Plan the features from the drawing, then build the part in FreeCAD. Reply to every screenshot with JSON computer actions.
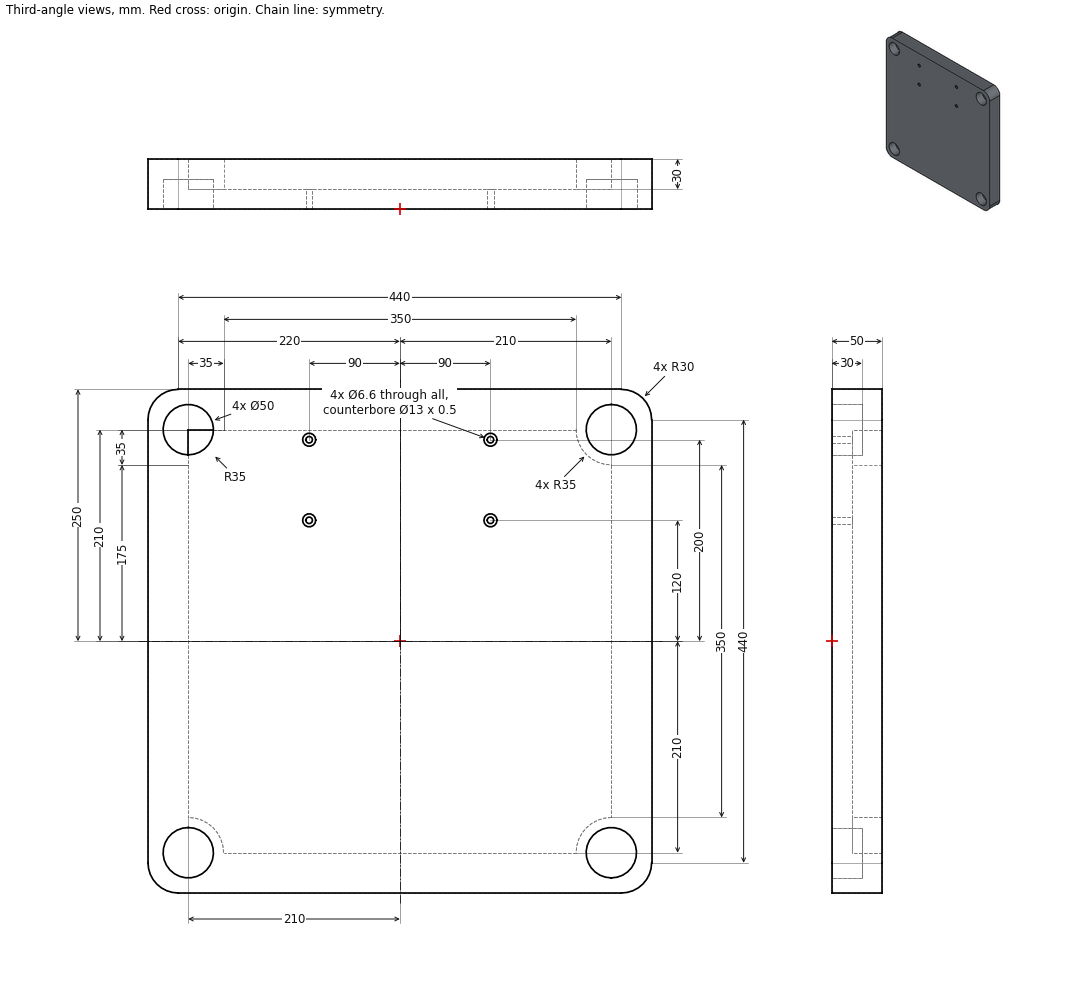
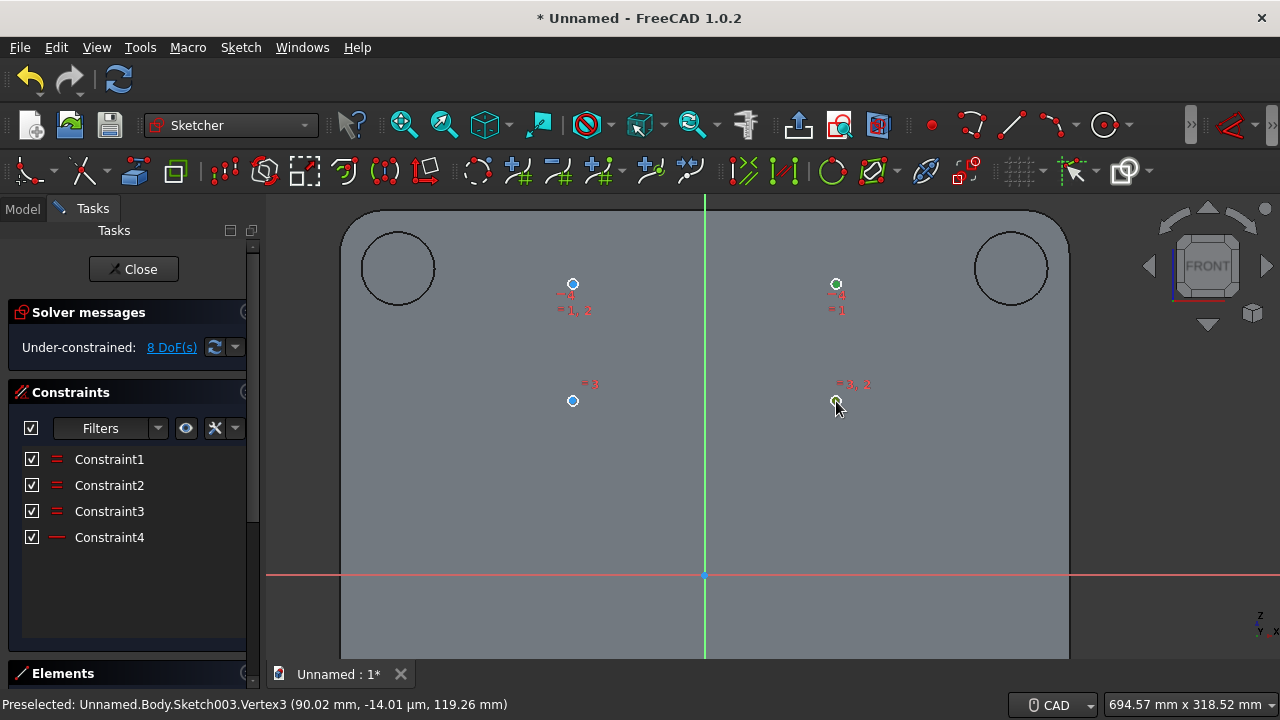
{"action": "key", "text": "v"}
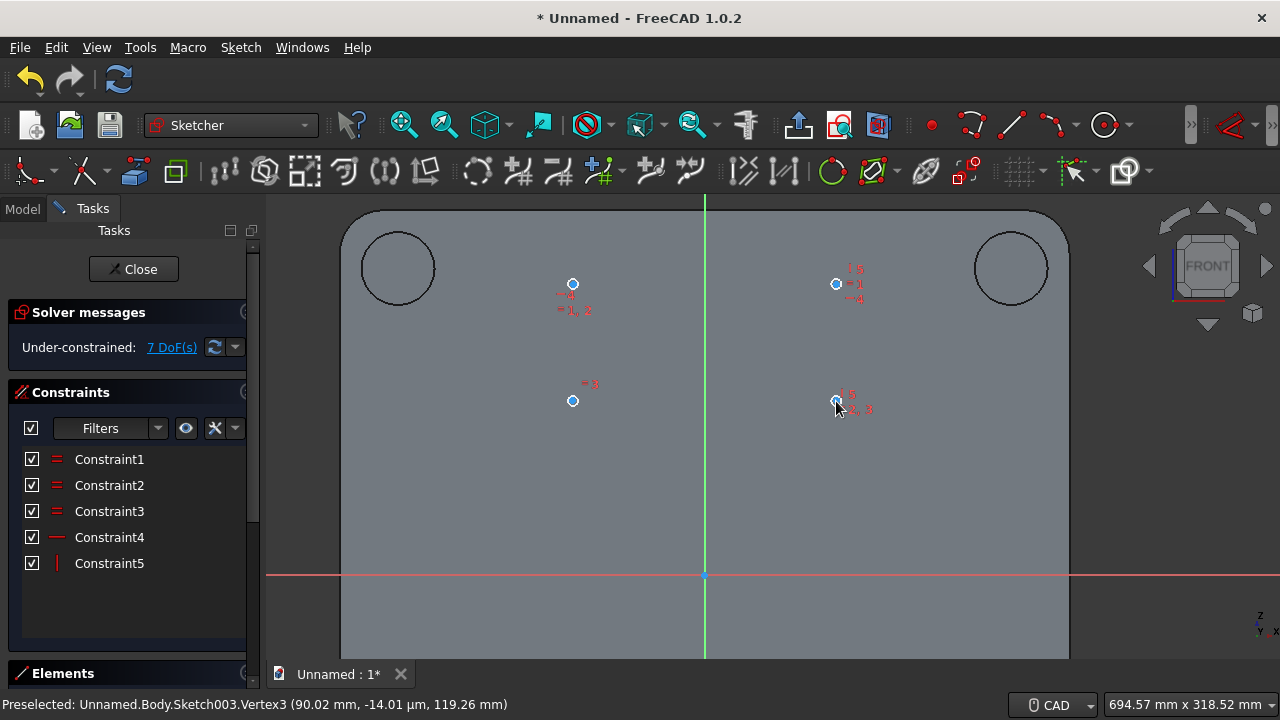
{"action": "left_click", "coordinate": [573, 284]}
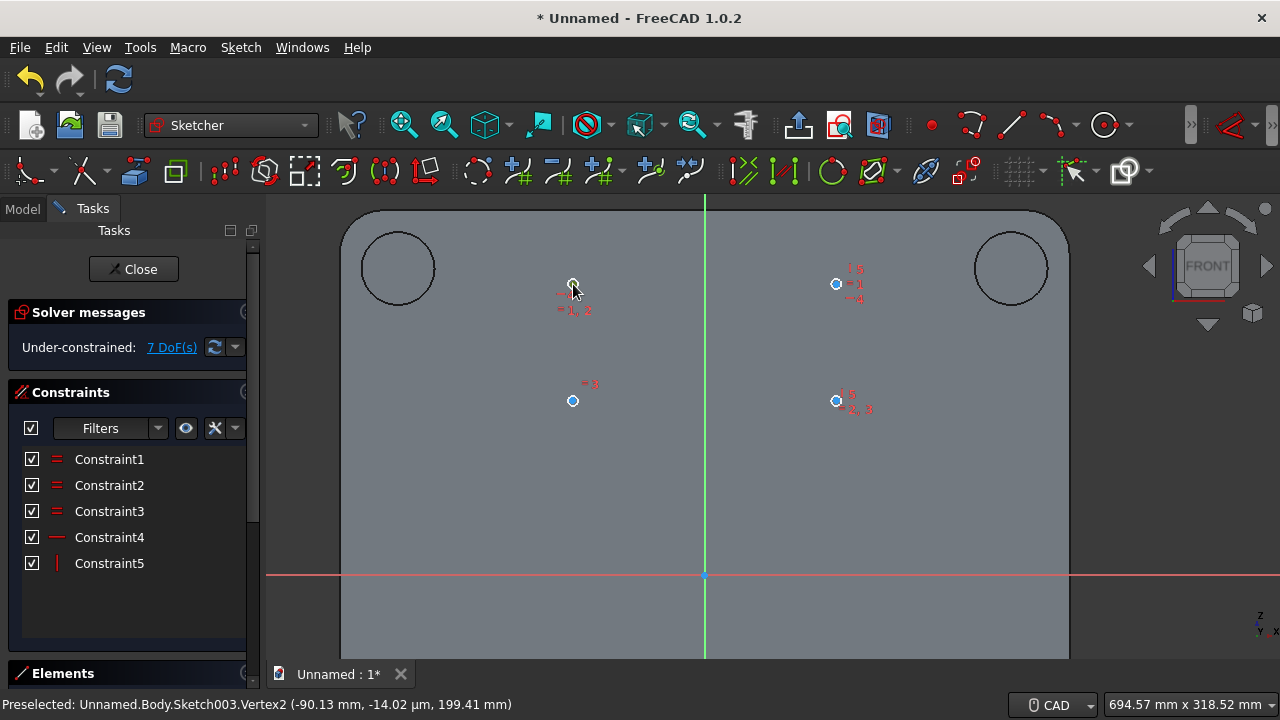
{"action": "left_click", "coordinate": [573, 401]}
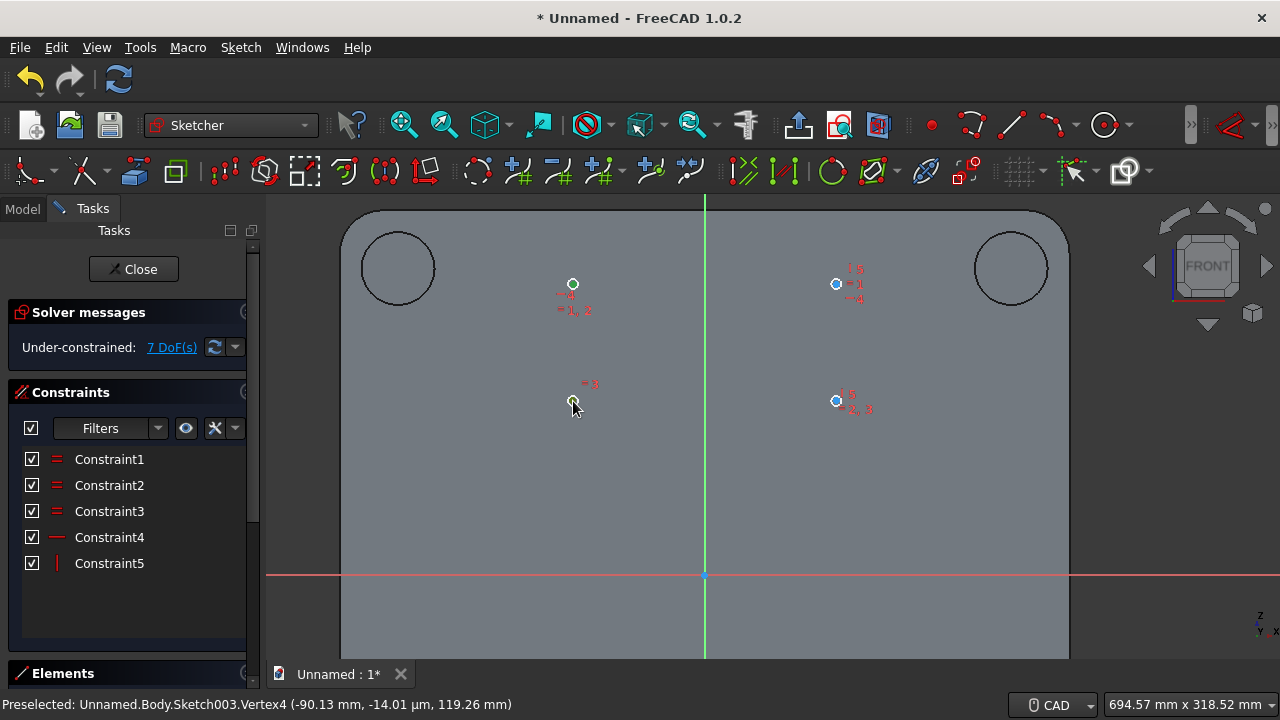
{"action": "key", "text": "v"}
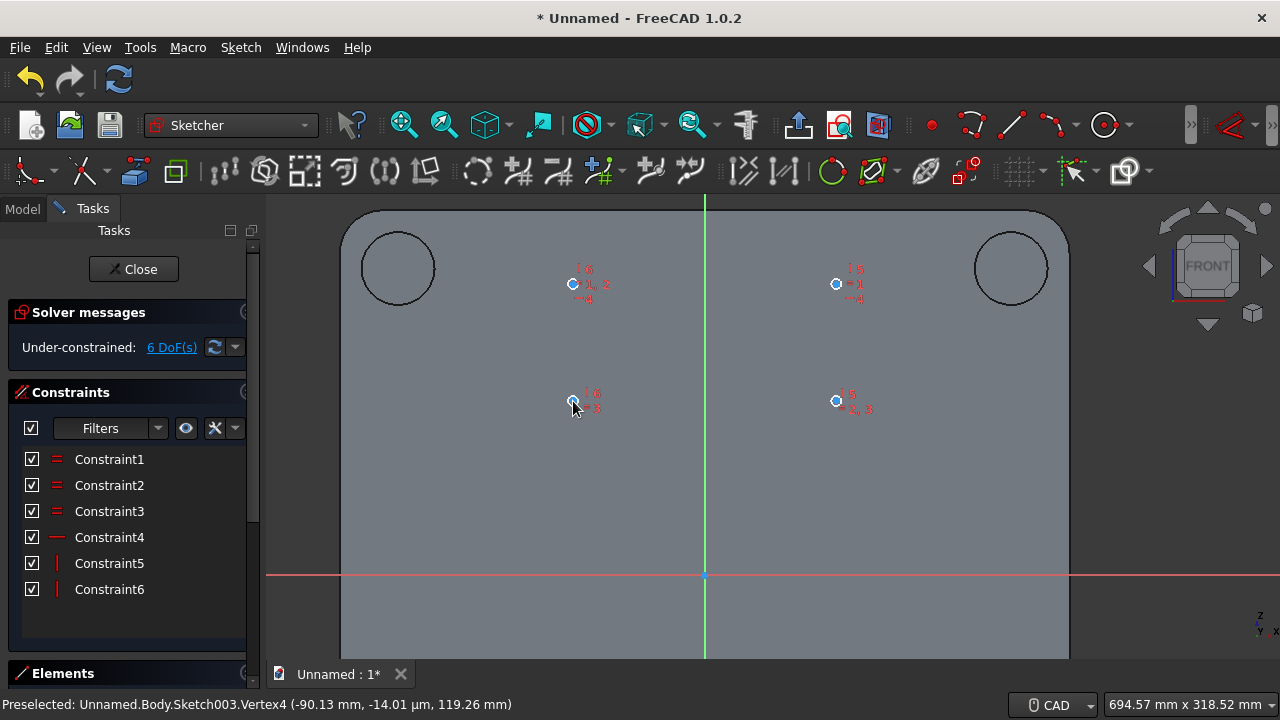
{"action": "left_click", "coordinate": [836, 401]}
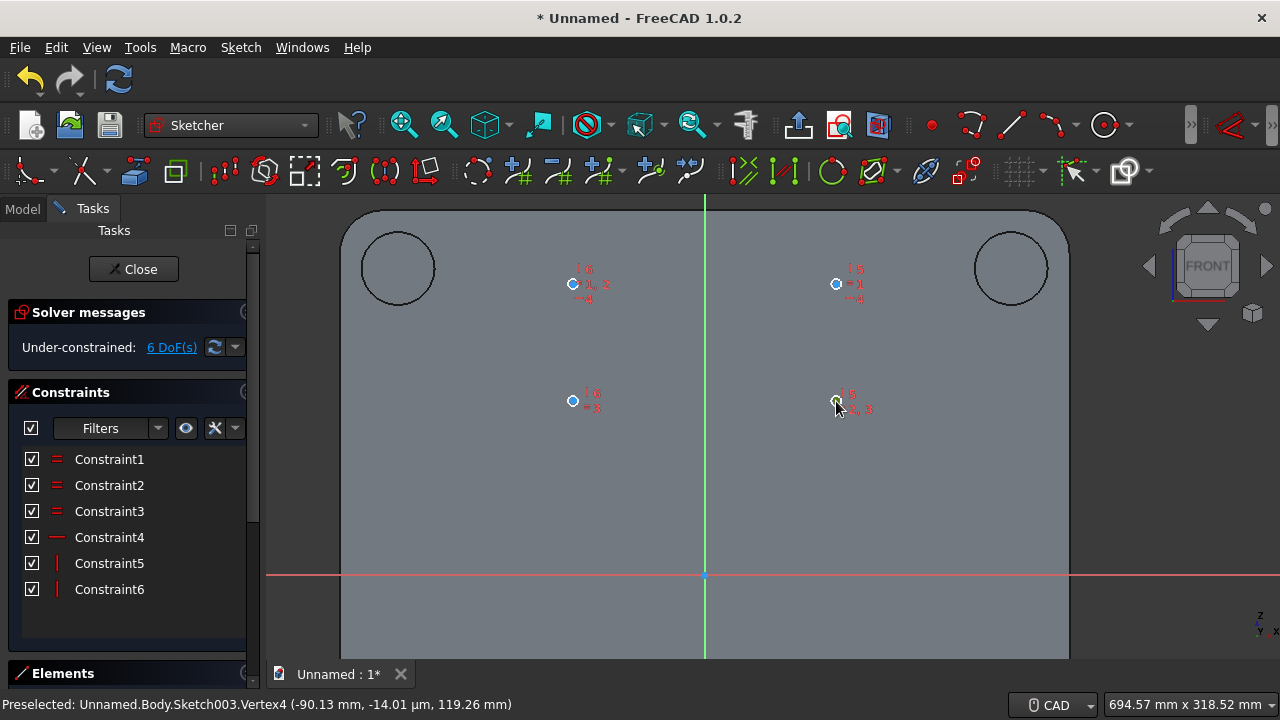
{"action": "left_click", "coordinate": [573, 401]}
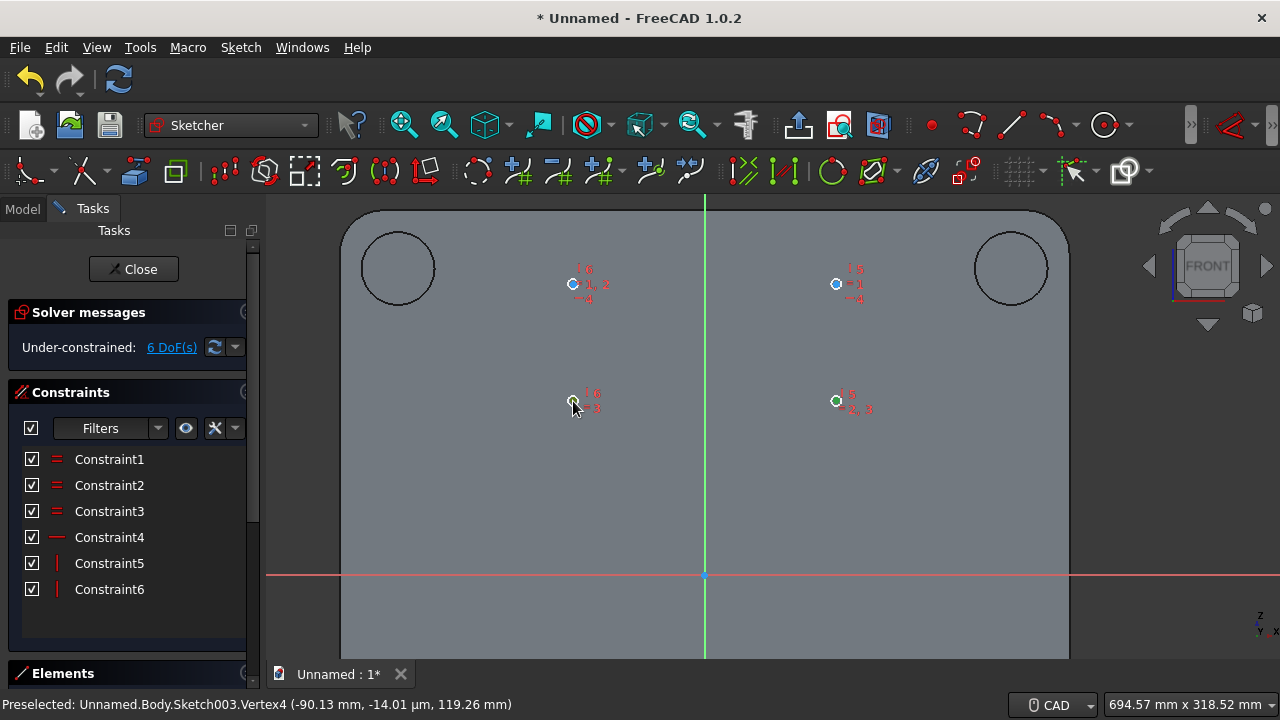
{"action": "key", "text": "h"}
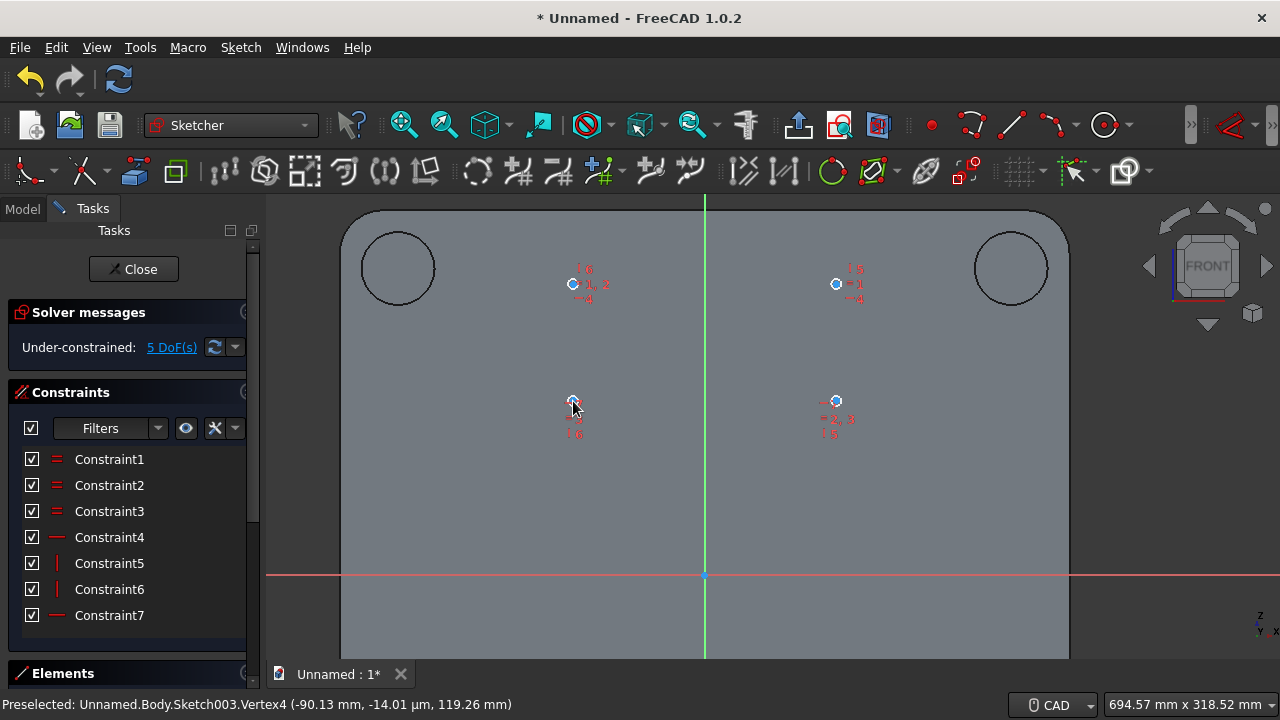
{"action": "key", "text": "d"}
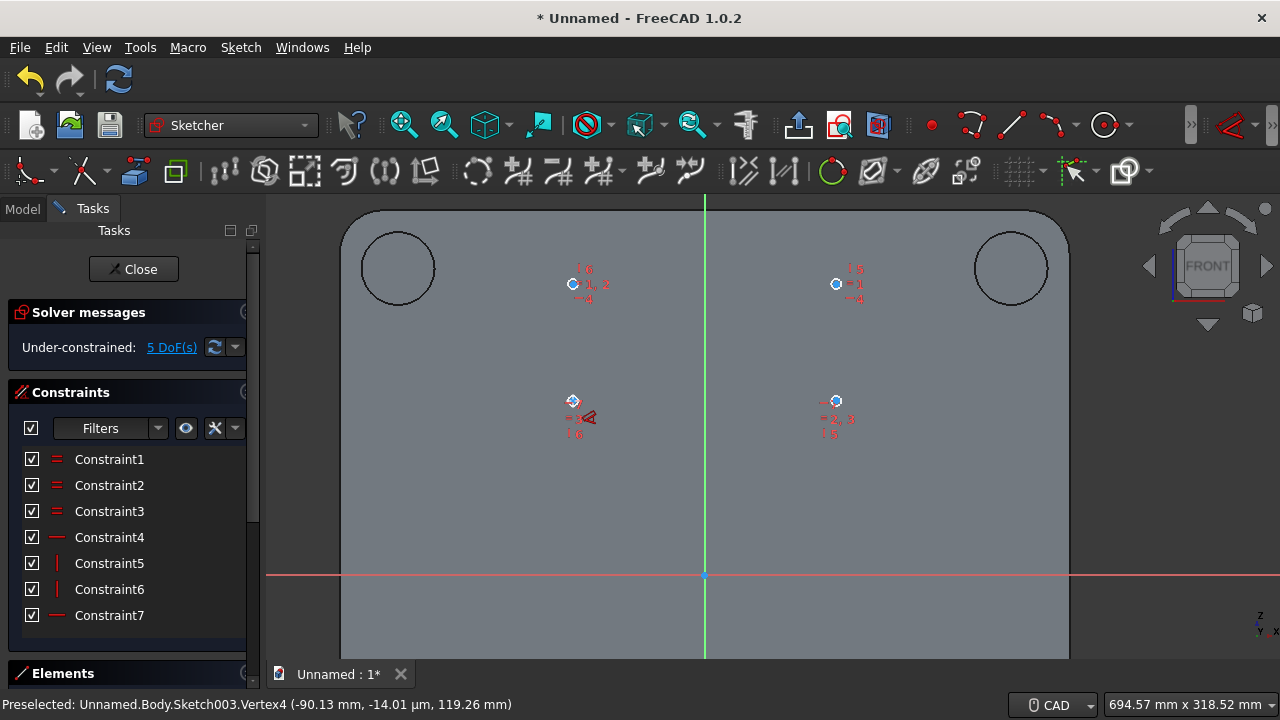
{"action": "scroll", "coordinate": [836, 279], "scroll_direction": "up", "scroll_amount": 8}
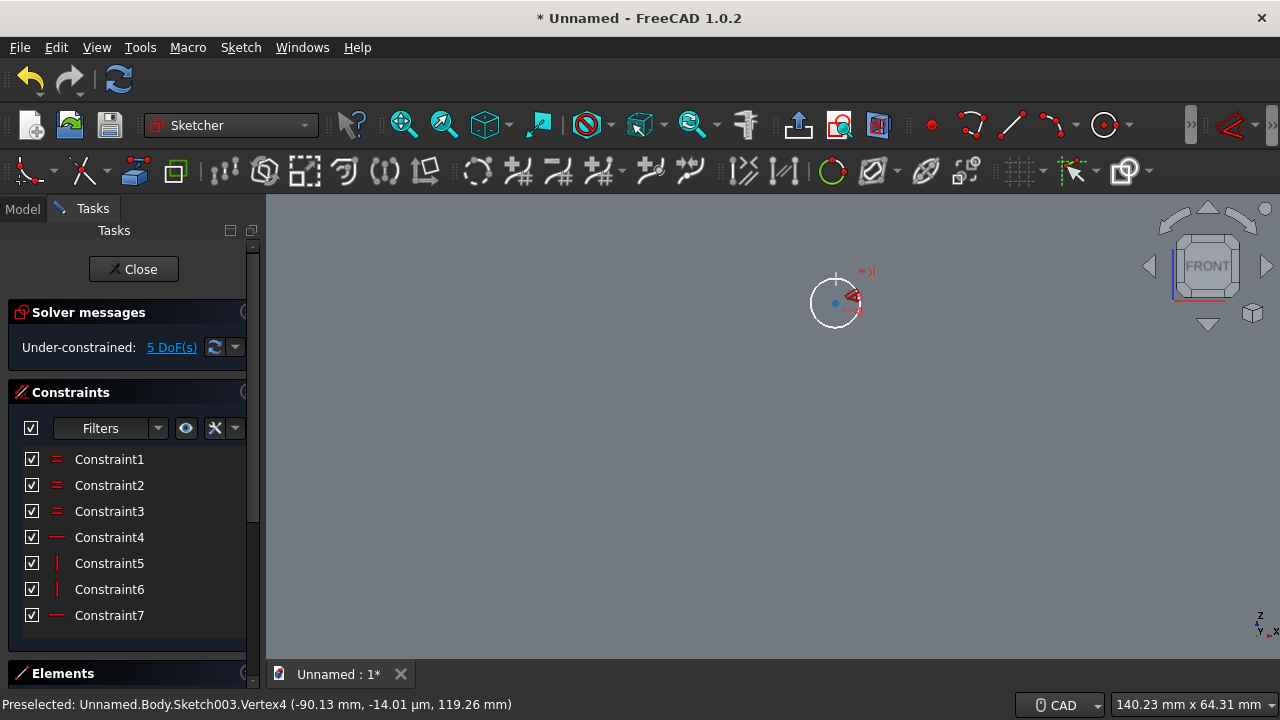
{"action": "left_click", "coordinate": [836, 279]}
{"action": "left_click", "coordinate": [837, 247]}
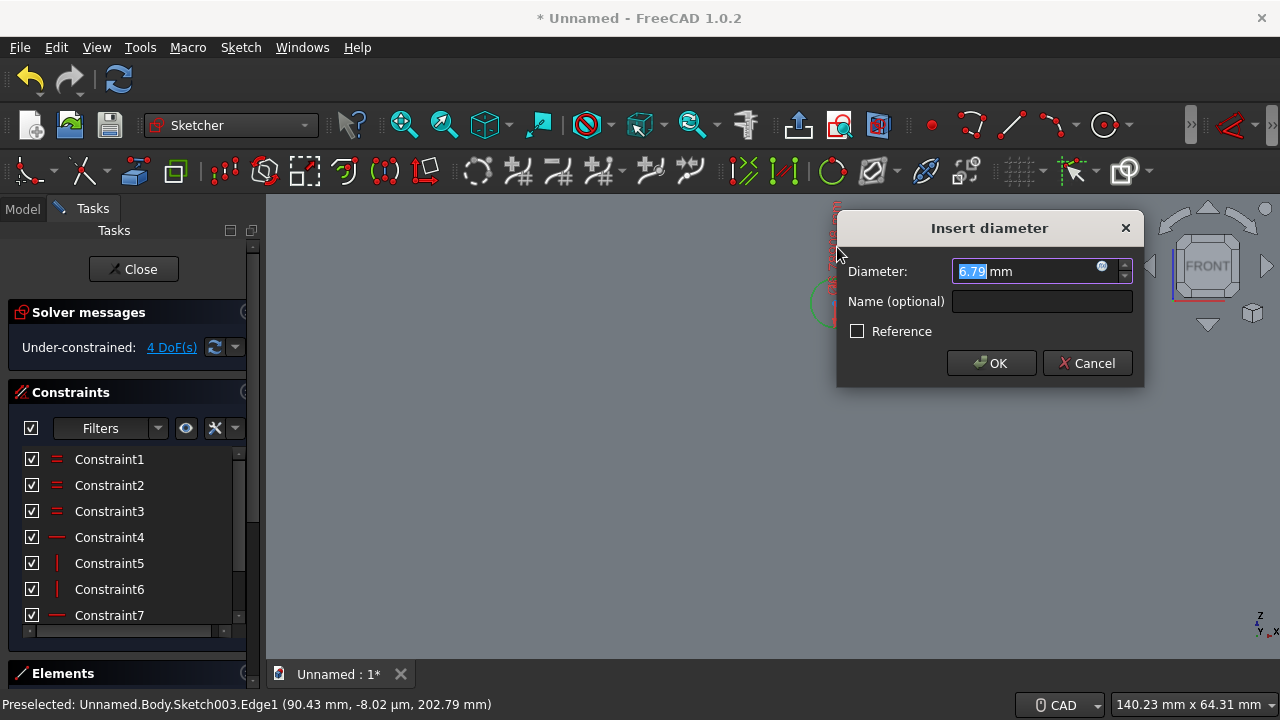
{"action": "type", "text": "6.6"}
{"action": "key", "text": "Return"}